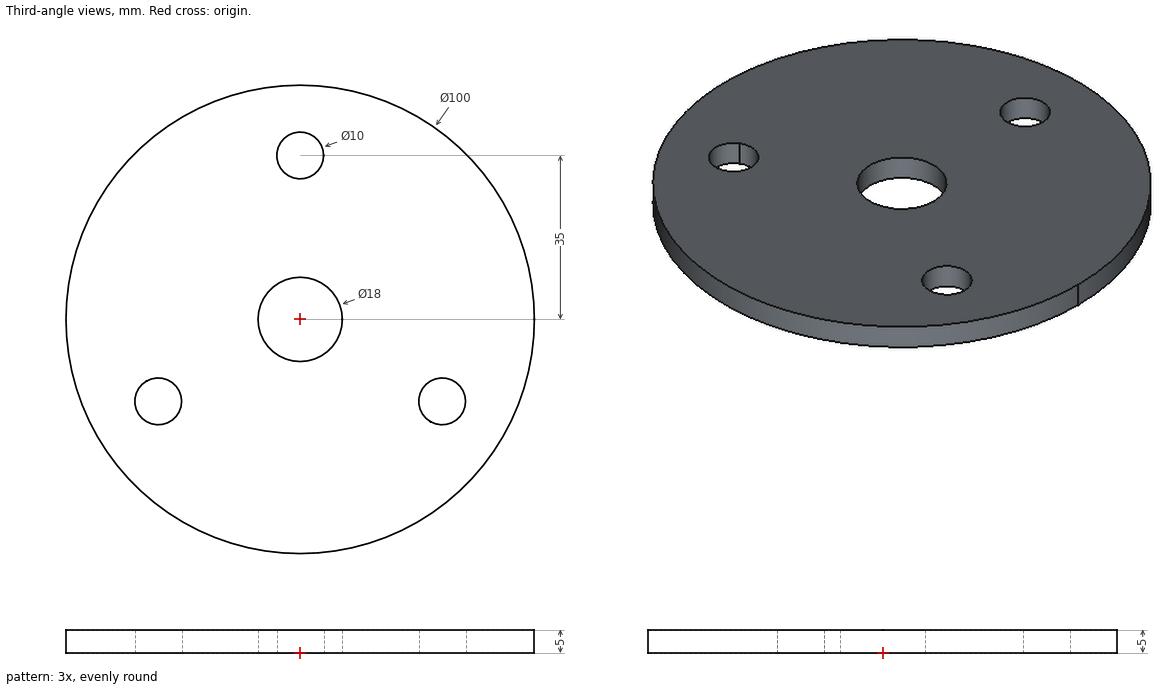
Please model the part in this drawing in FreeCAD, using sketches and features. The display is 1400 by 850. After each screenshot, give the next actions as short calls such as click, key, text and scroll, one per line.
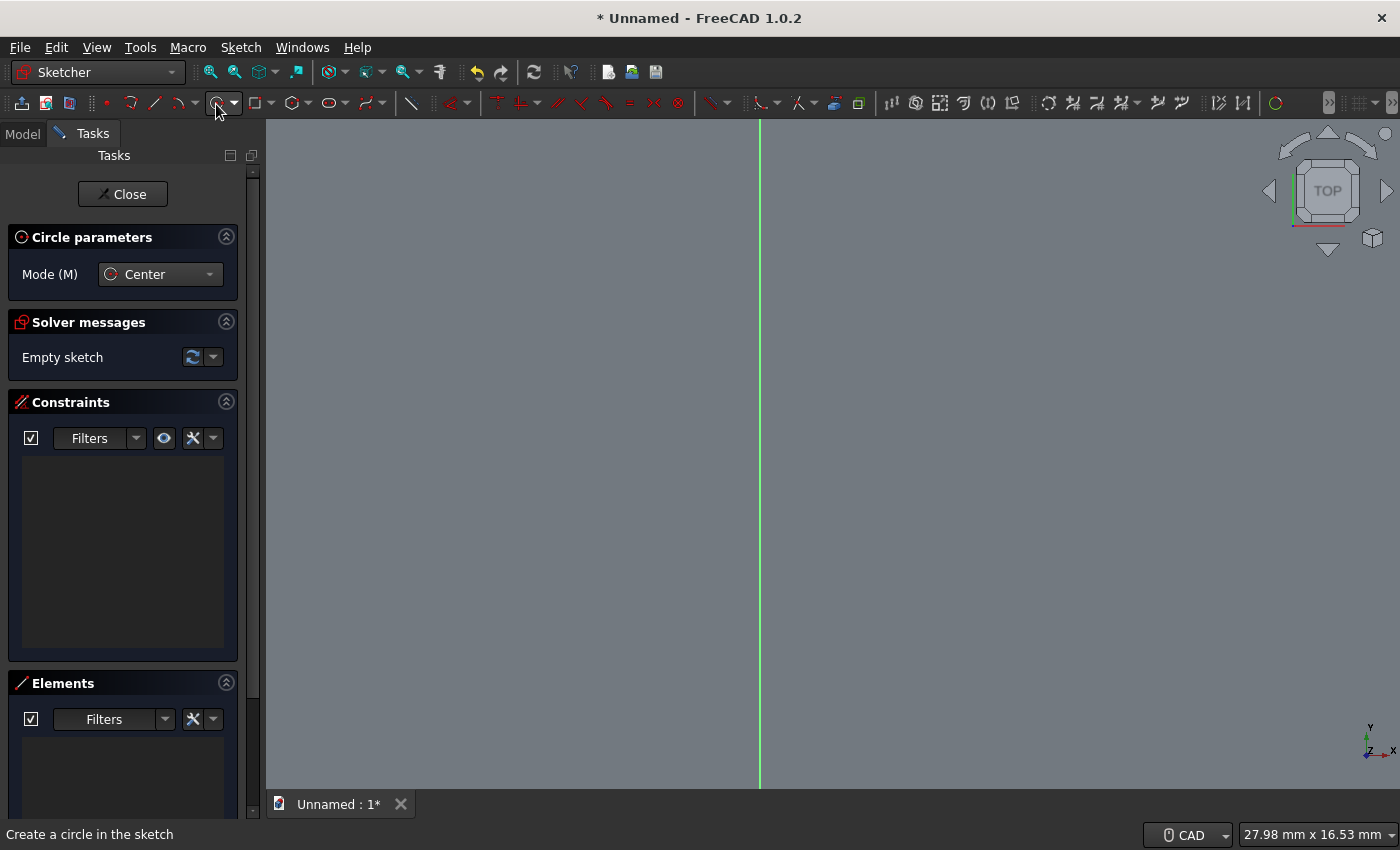
click(760, 454)
click(903, 311)
key(Escape)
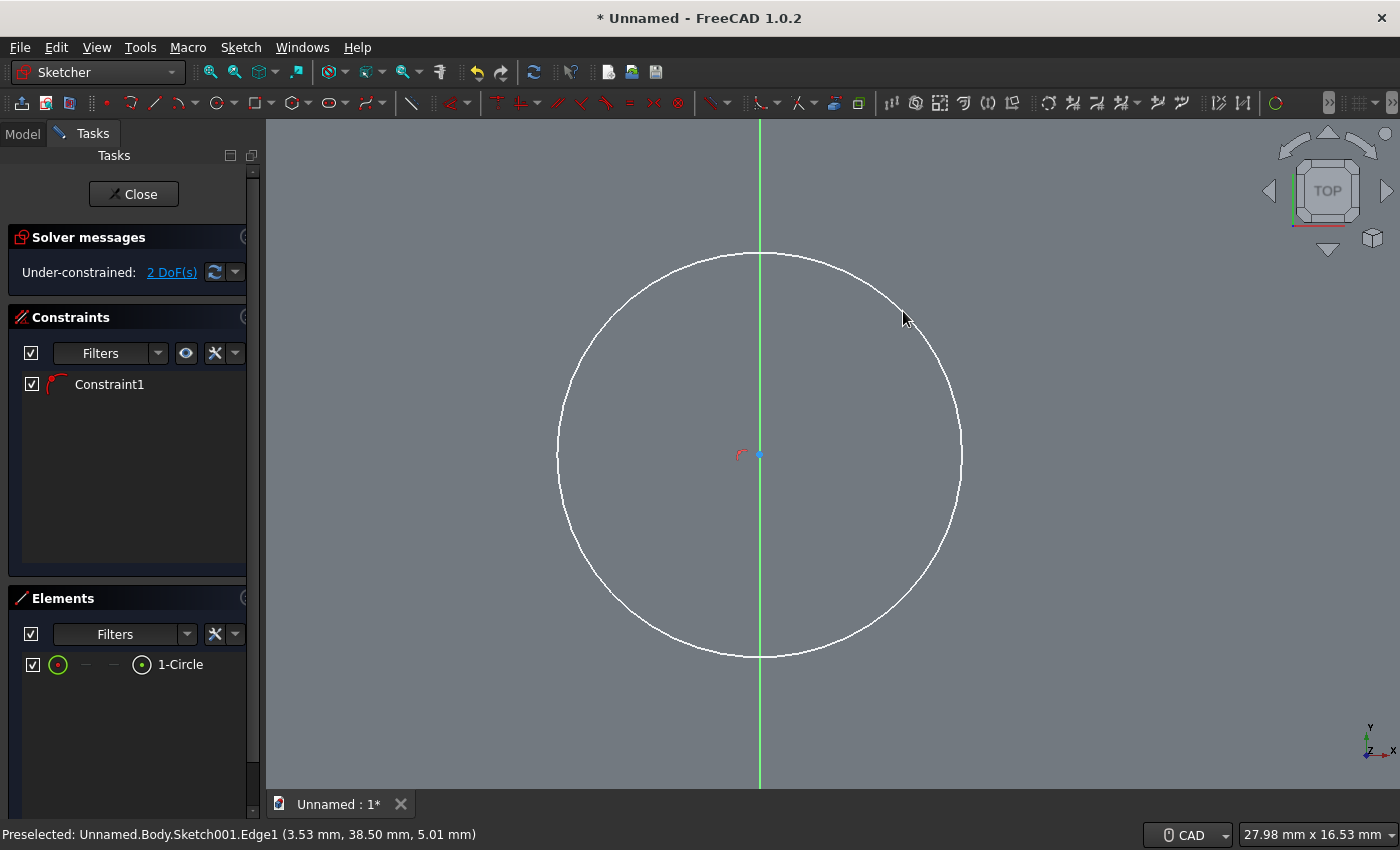
click(450, 104)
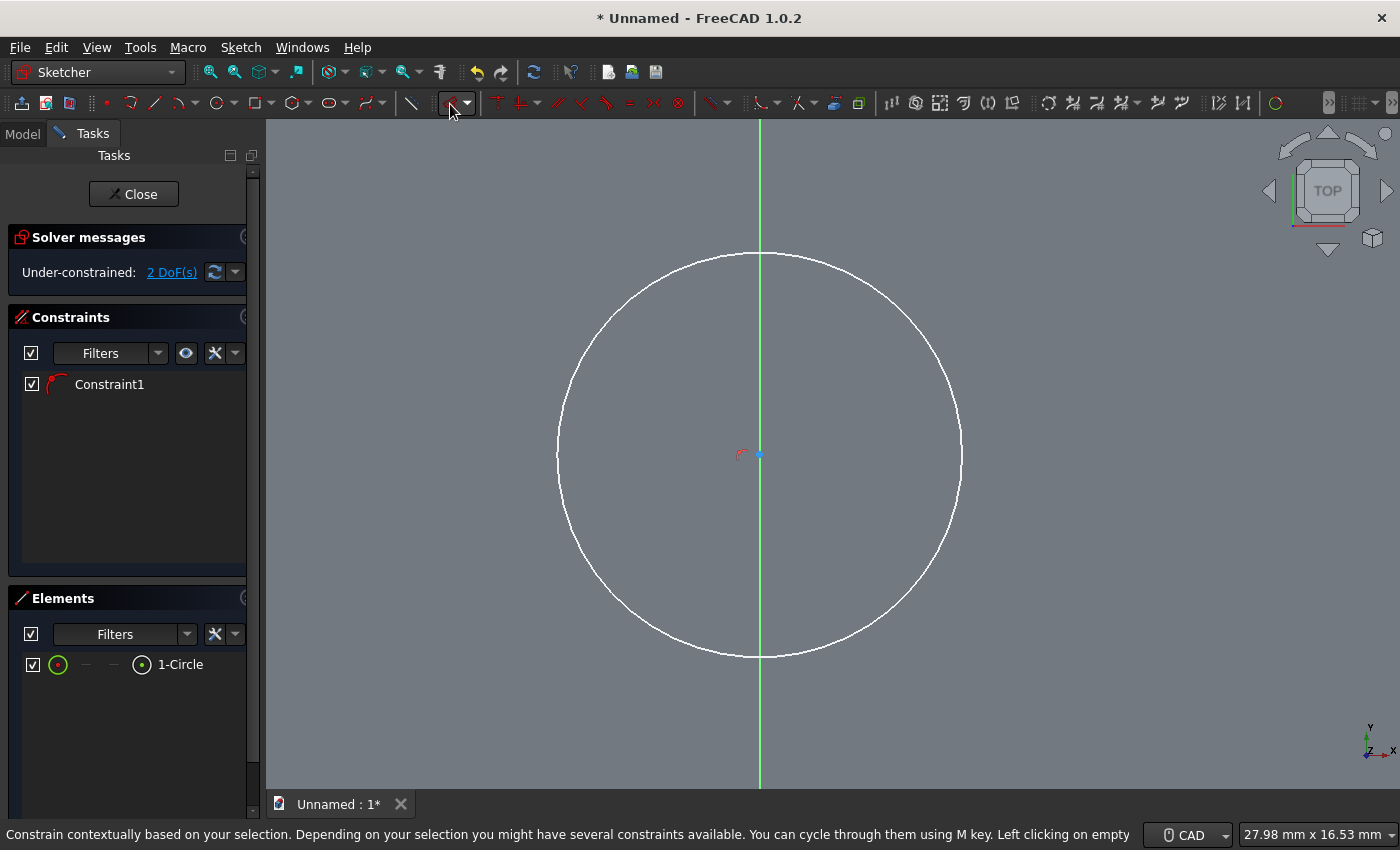
click(902, 311)
click(924, 288)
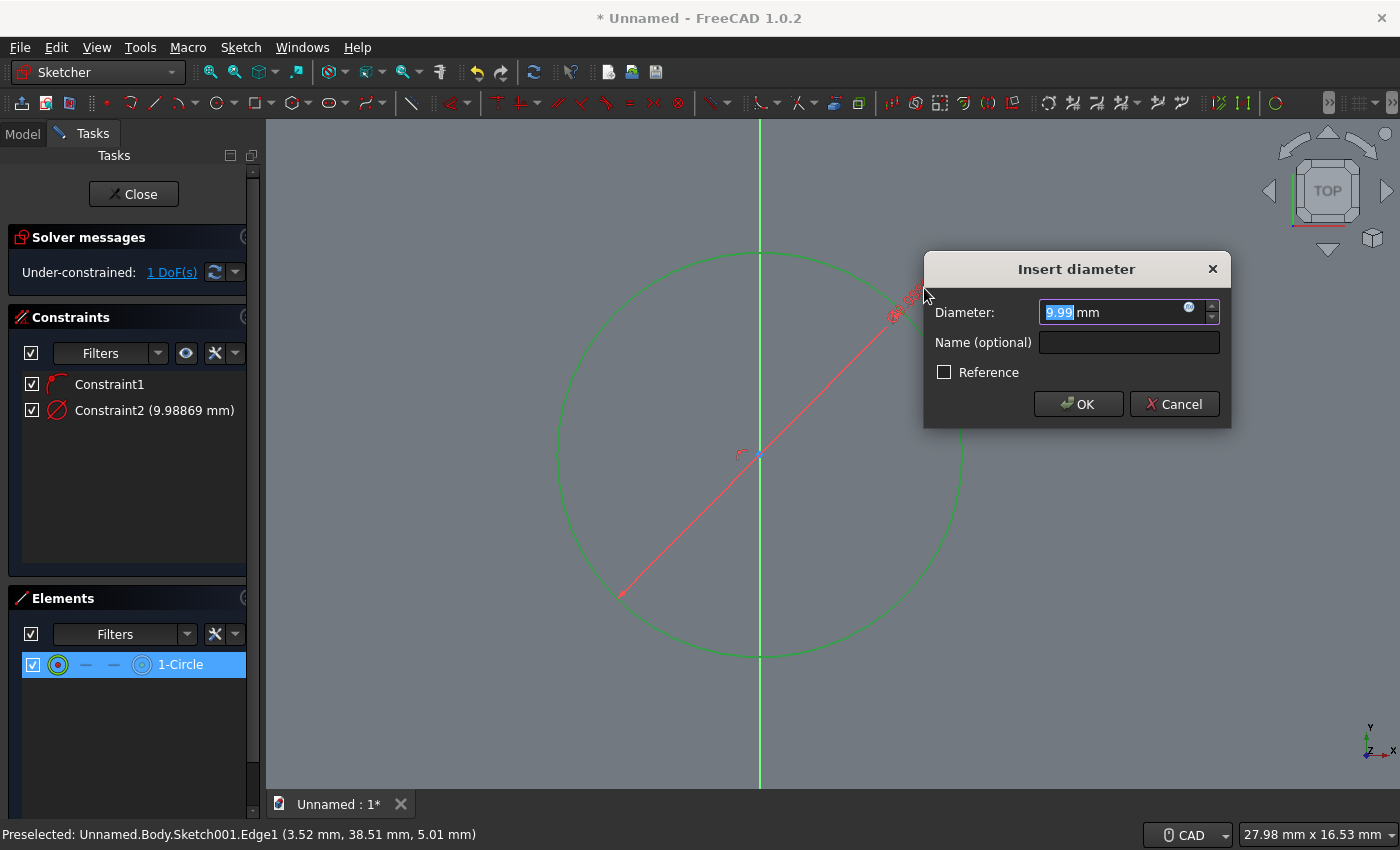
text(10)
key(Return)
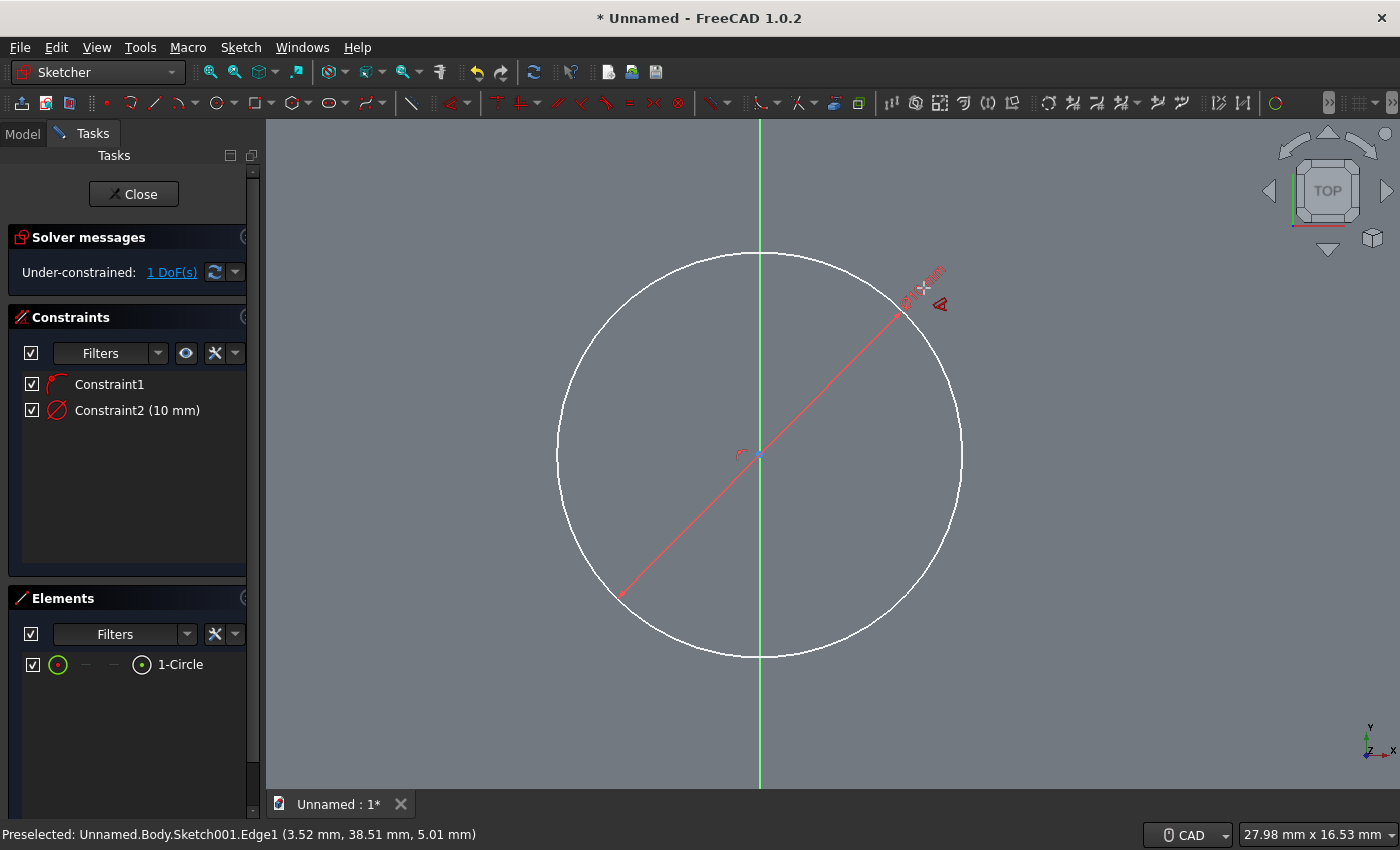
click(760, 455)
click(794, 608)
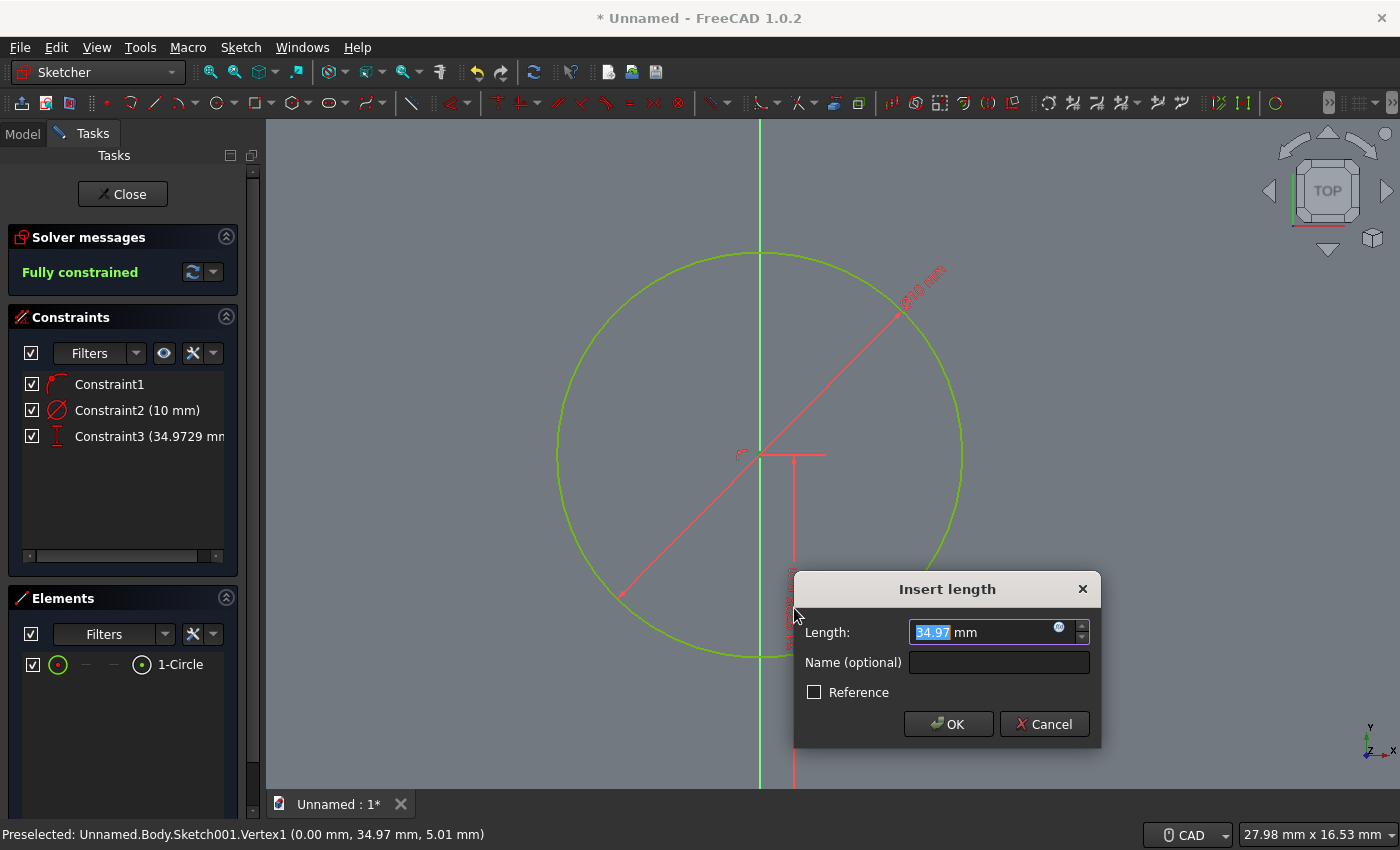
text(35)
key(Return)
key(Escape)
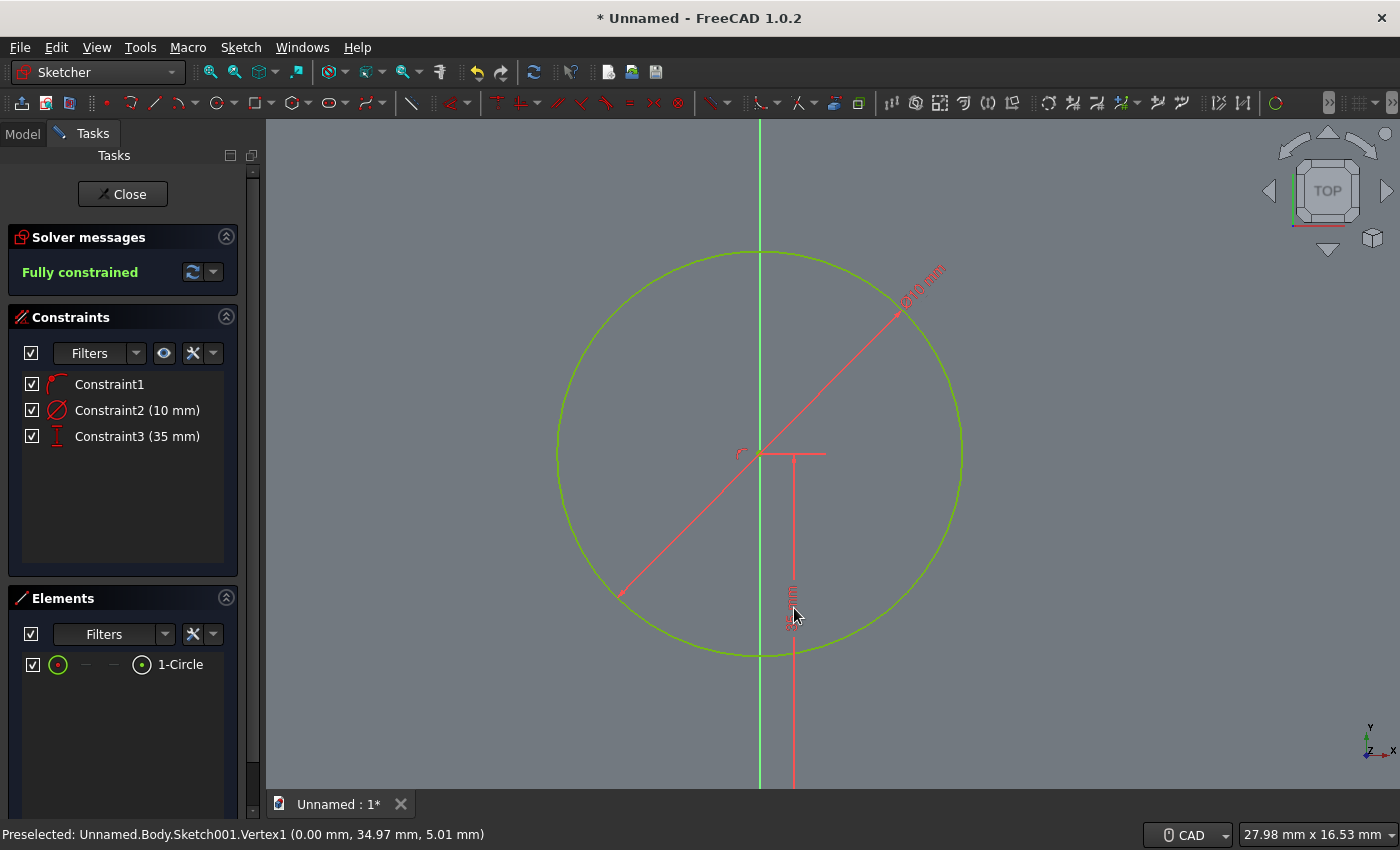
click(123, 194)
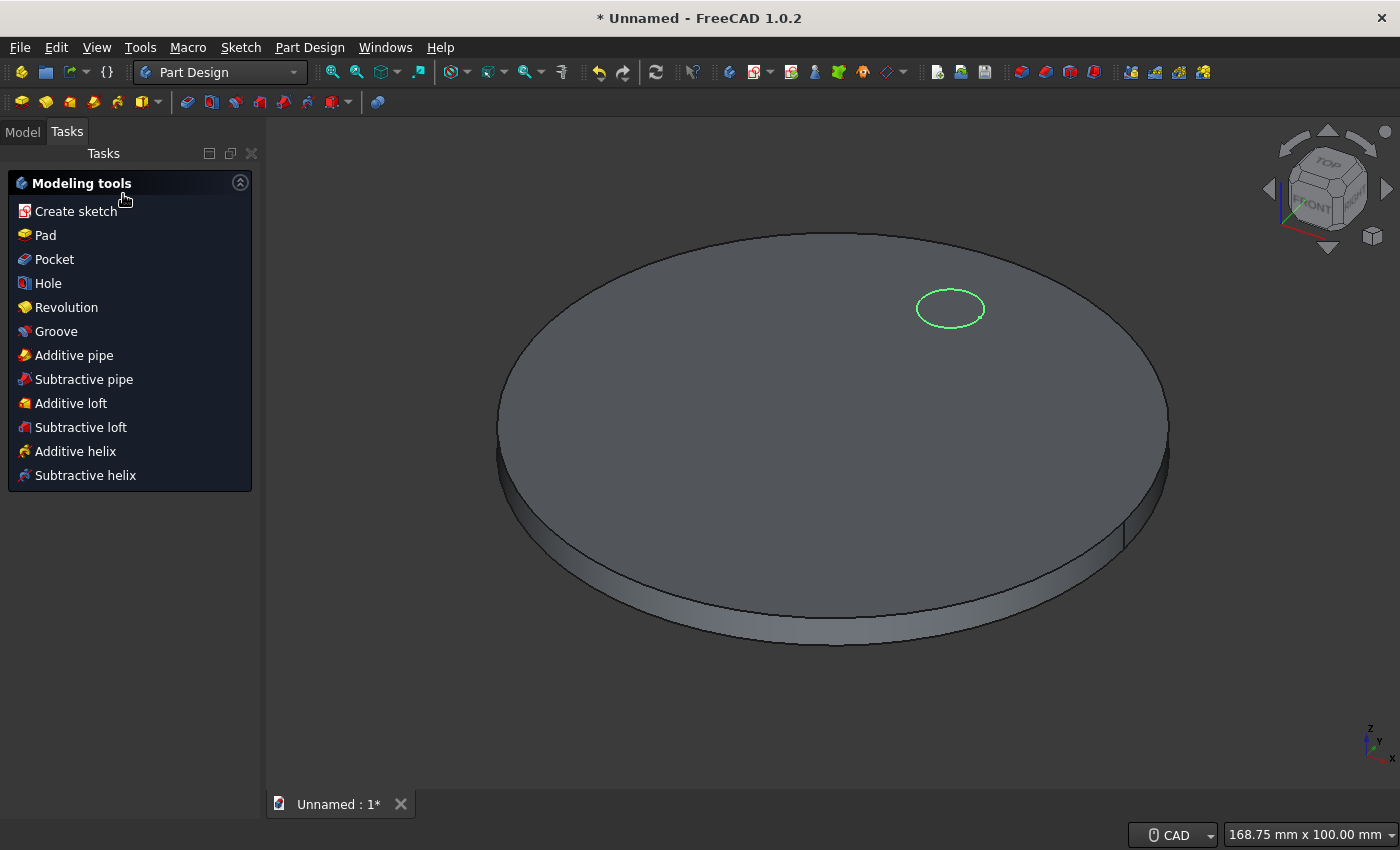
click(188, 102)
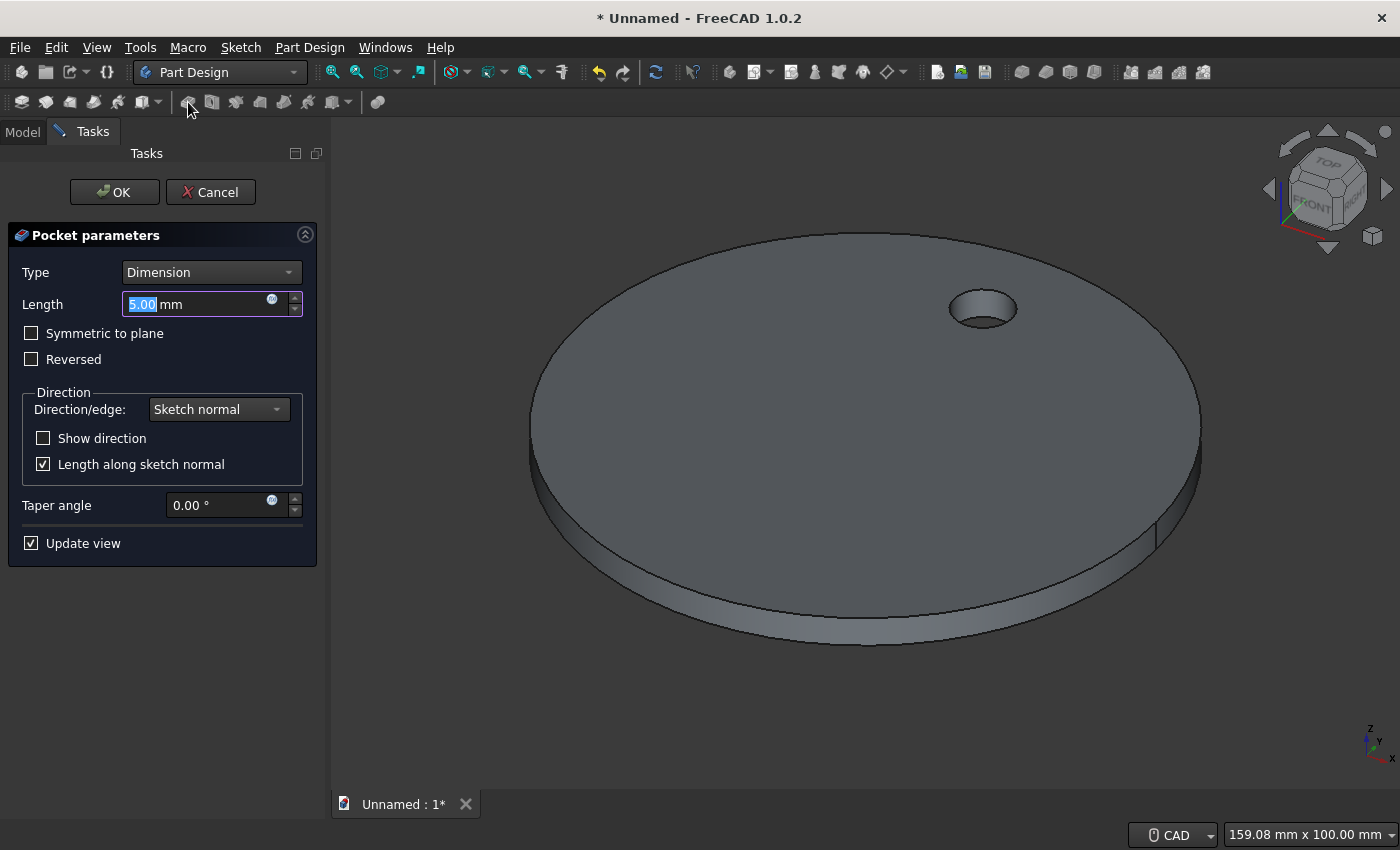
text(5)
key(Tab)